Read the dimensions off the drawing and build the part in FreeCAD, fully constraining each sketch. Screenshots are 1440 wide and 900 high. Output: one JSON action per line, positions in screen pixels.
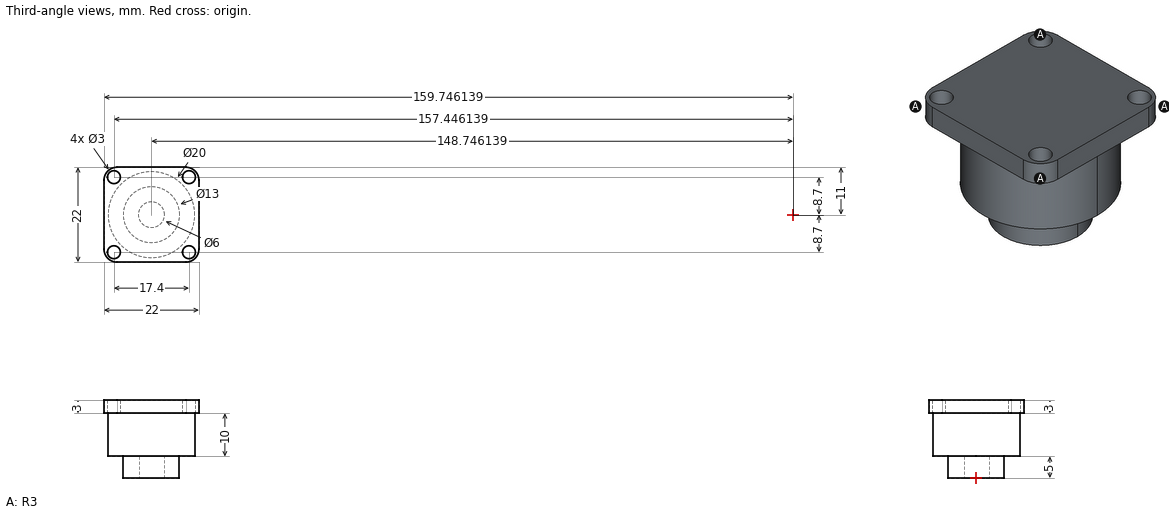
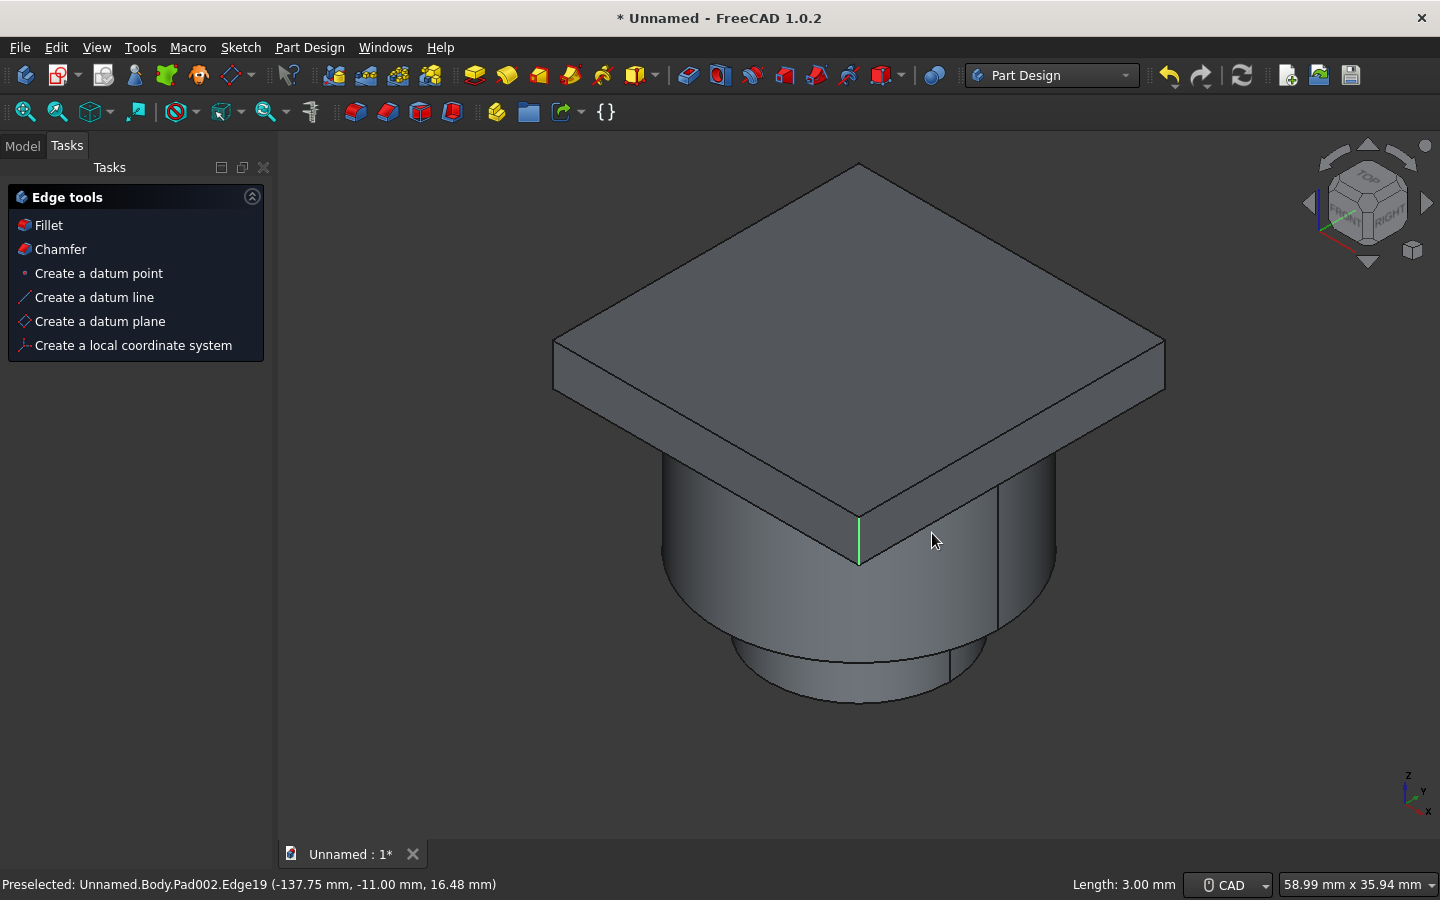
{"action": "key", "text": "2"}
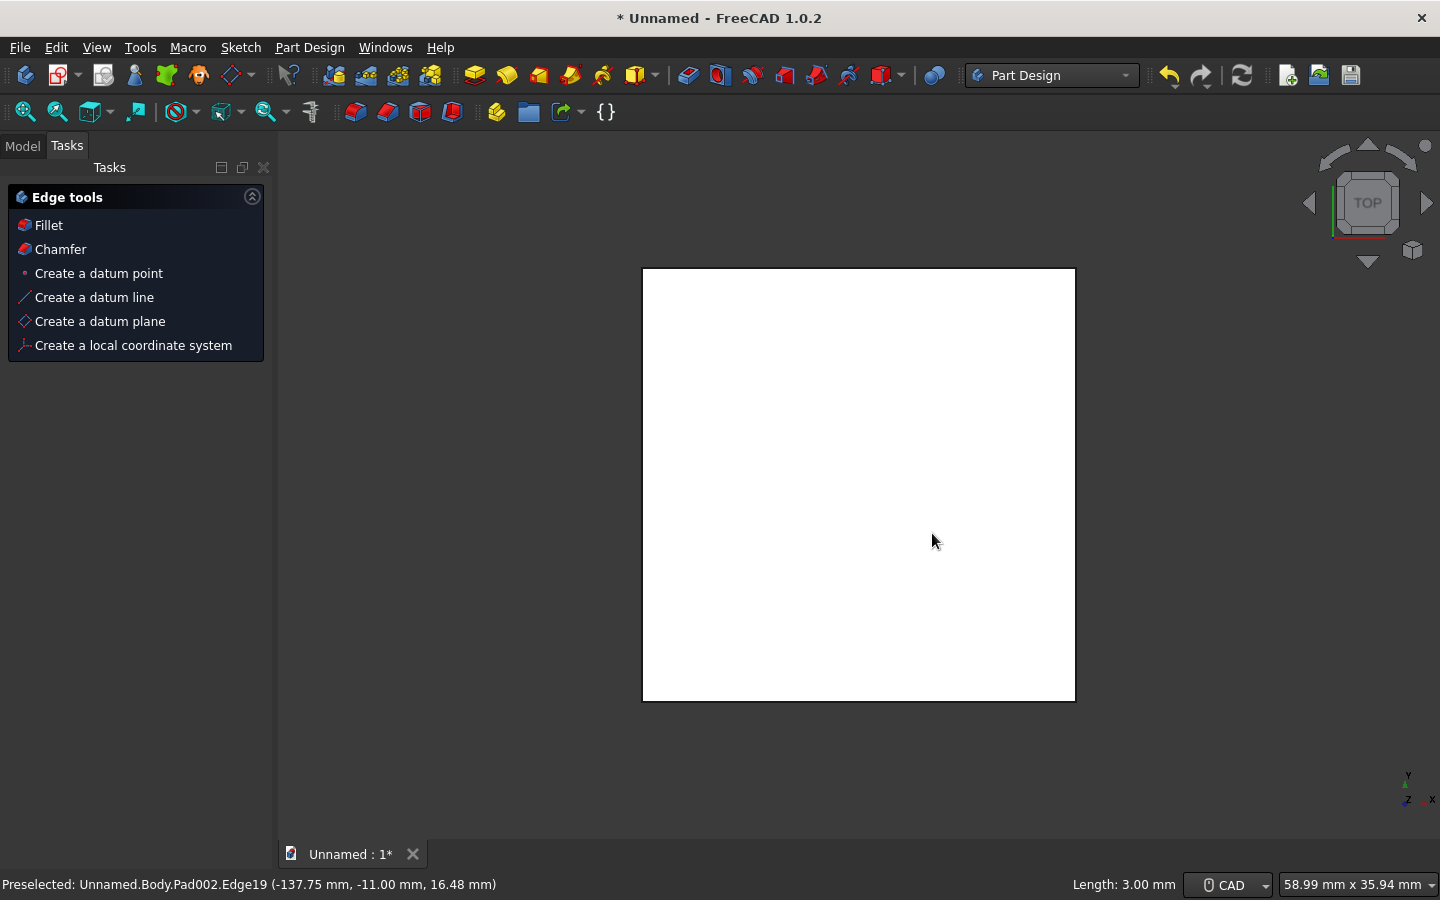
{"action": "key", "text": "1"}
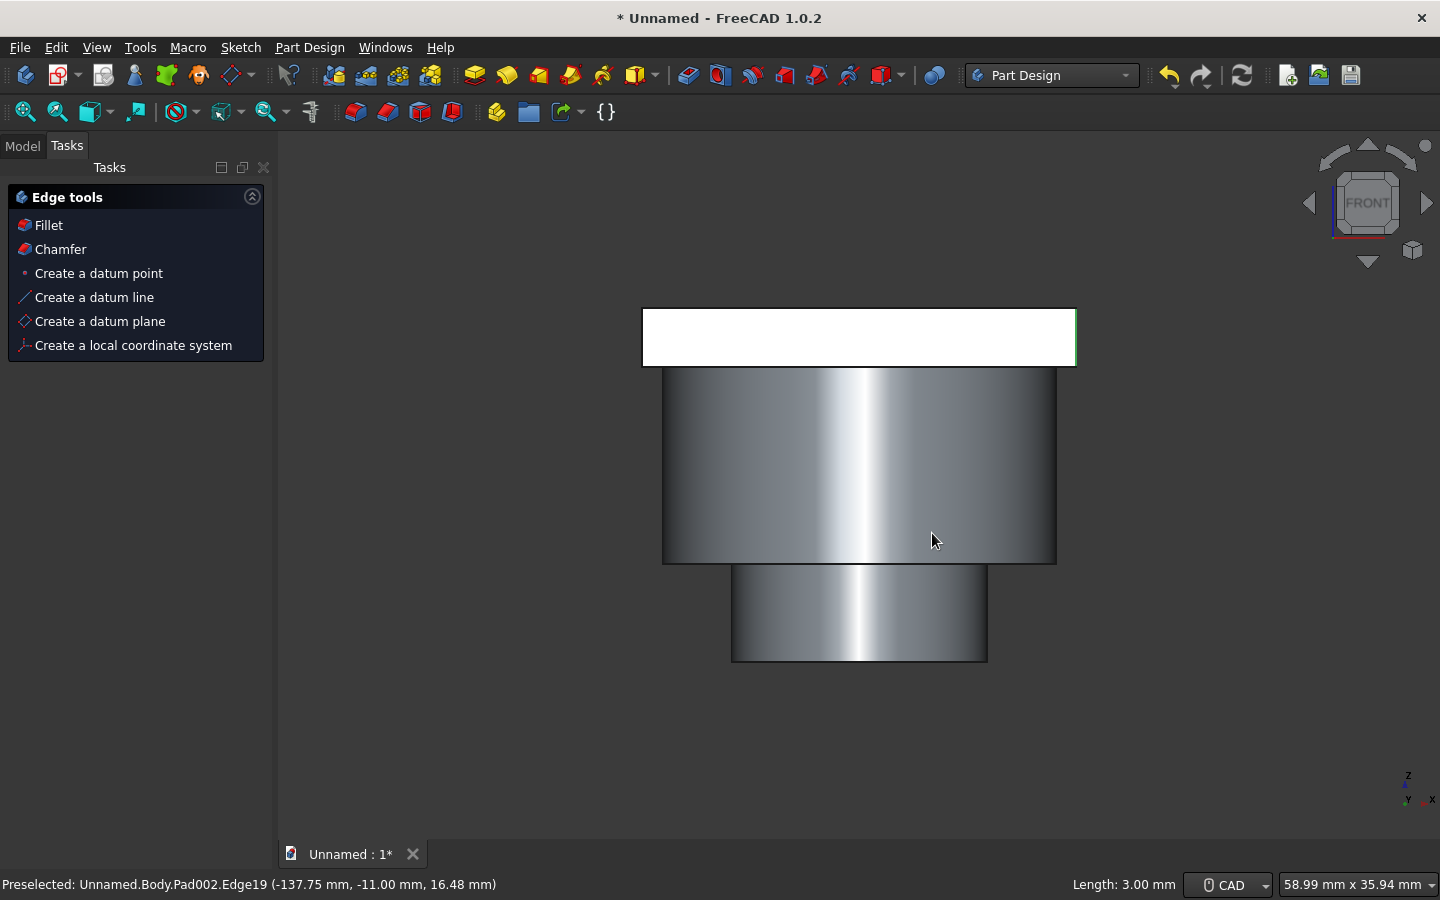
{"action": "left_click", "coordinate": [642, 336], "text": "ctrl"}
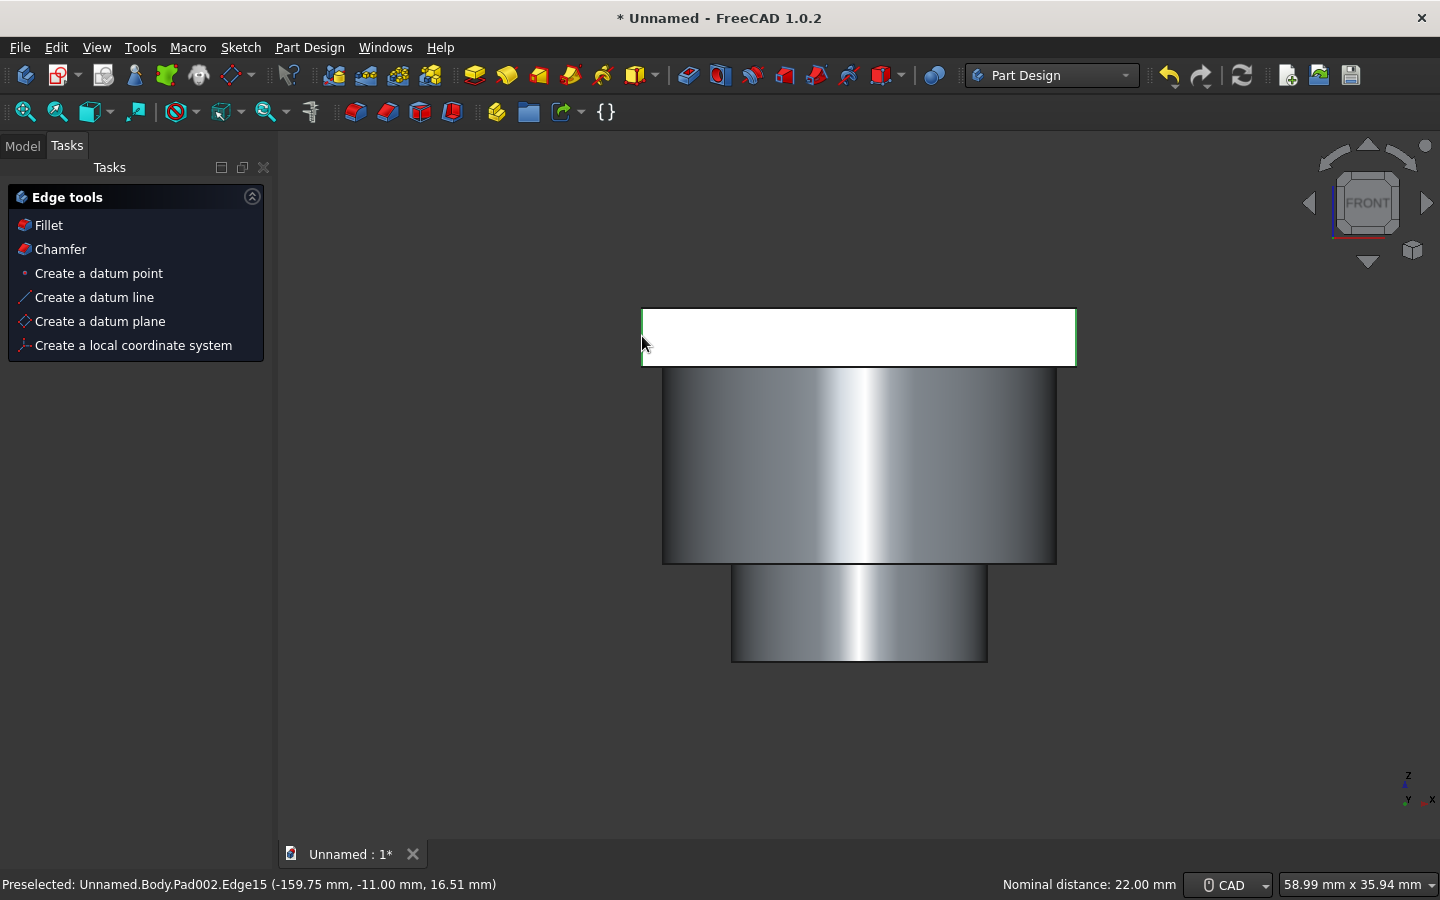
{"action": "key", "text": "3"}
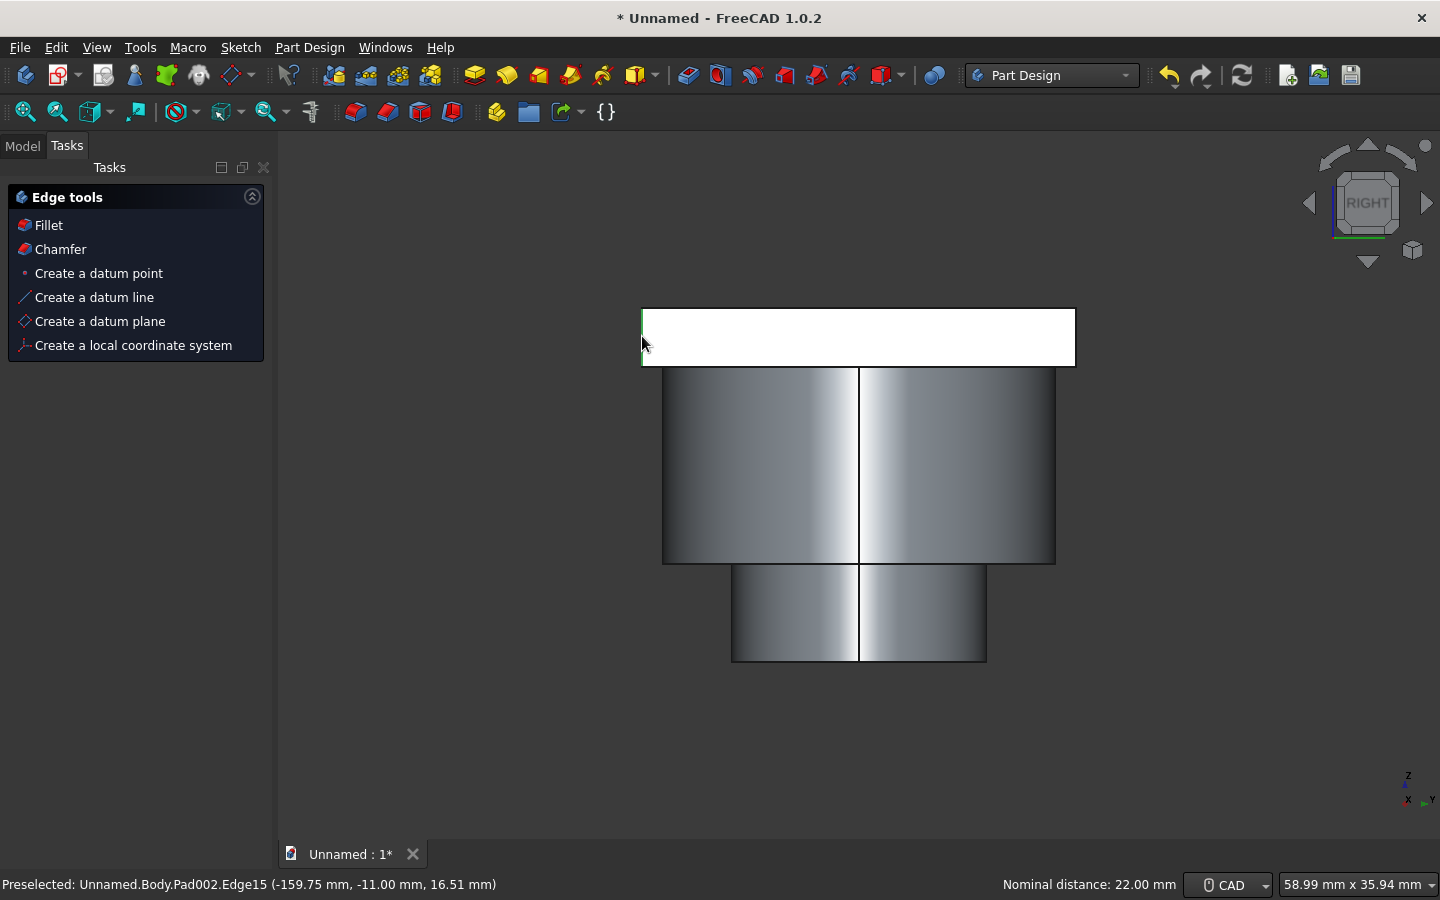
{"action": "left_click", "coordinate": [1076, 336], "text": "ctrl"}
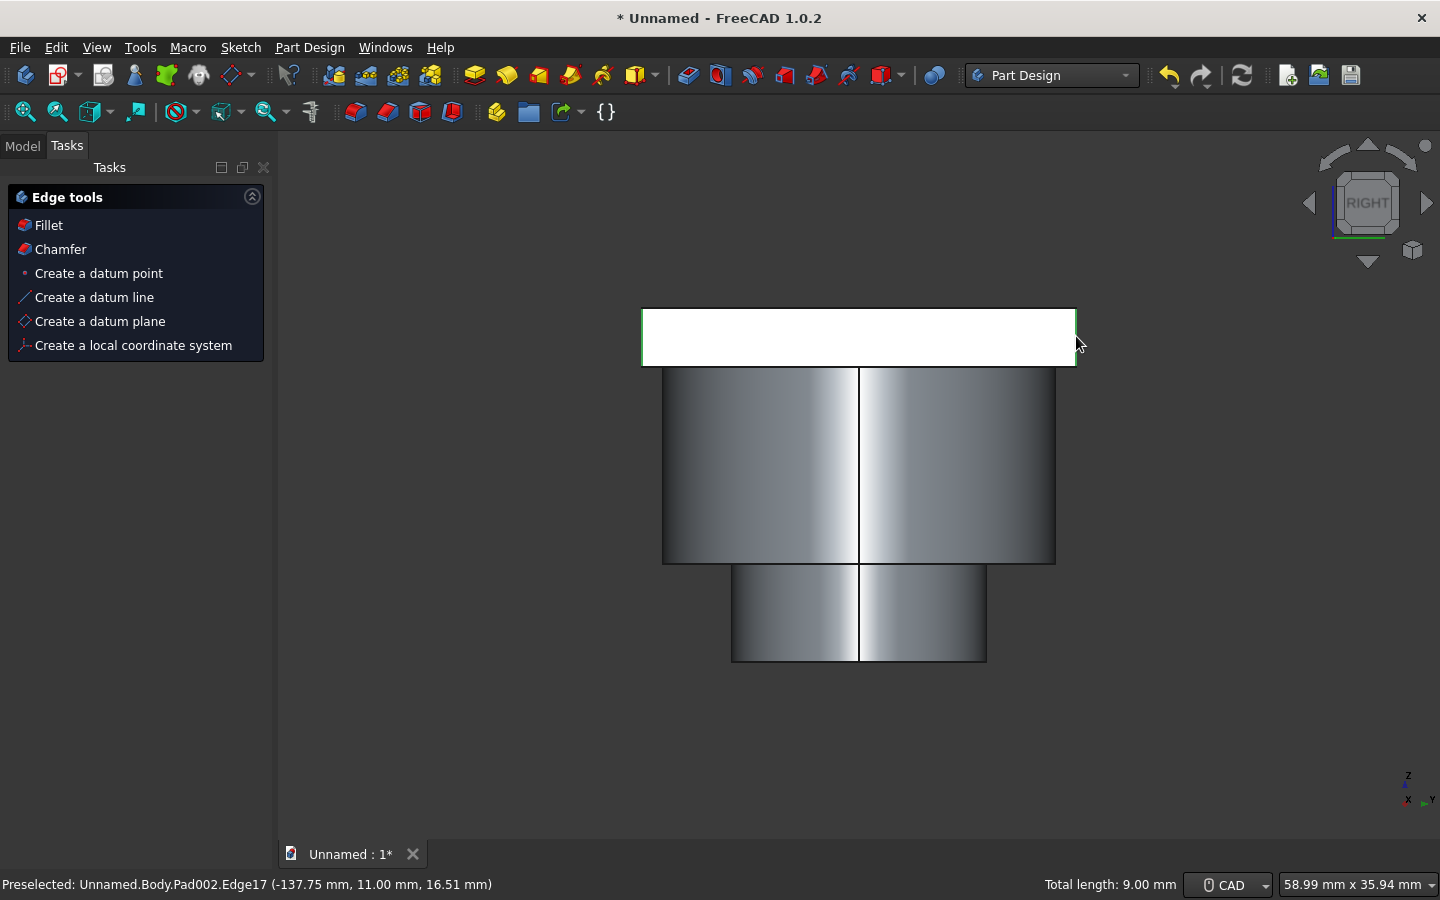
{"action": "key", "text": "5"}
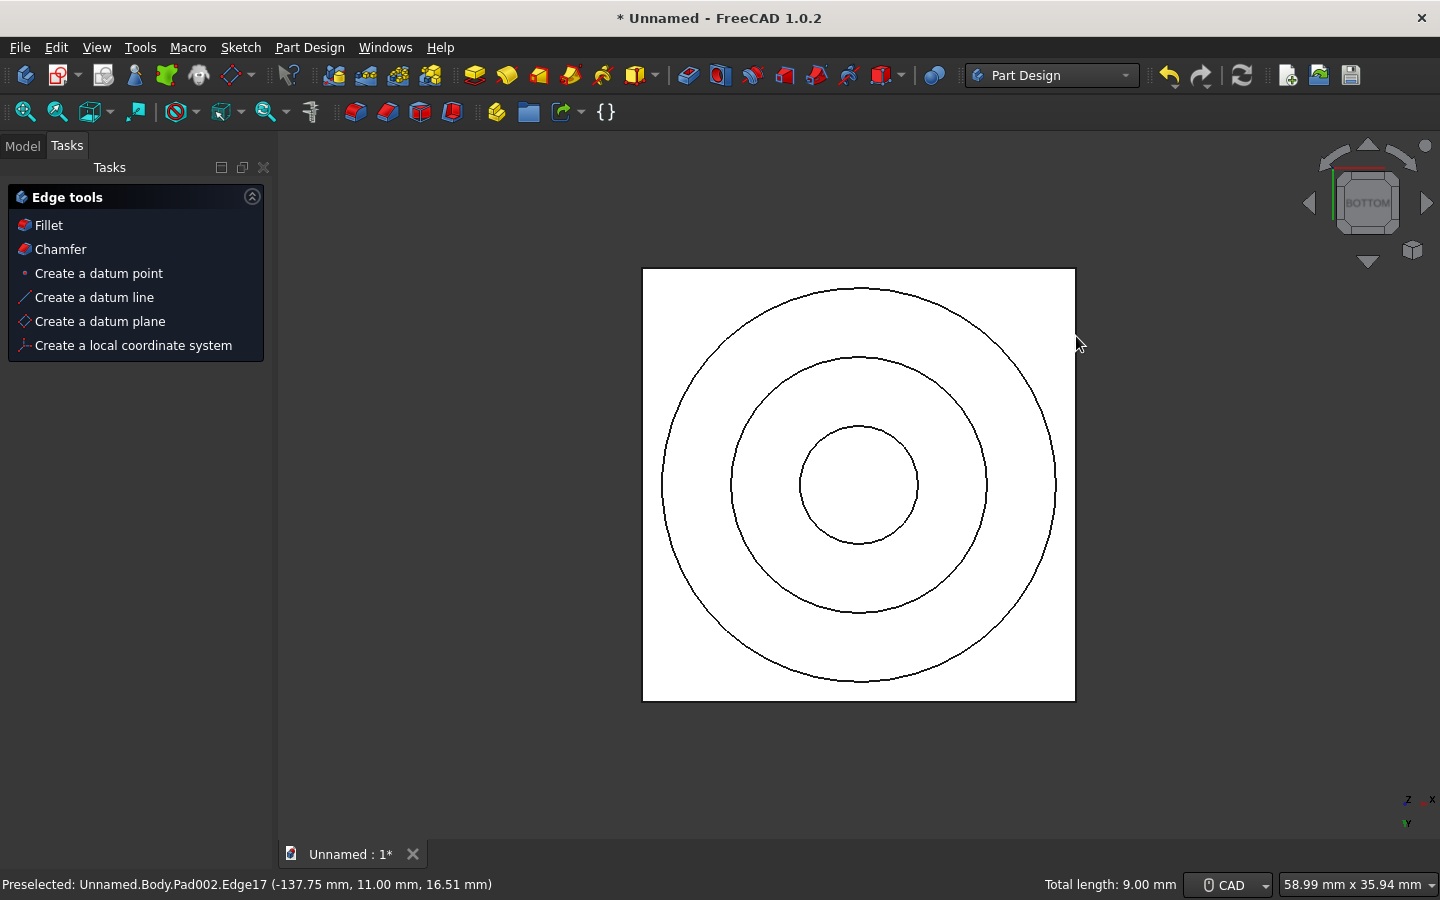
{"action": "key", "text": "4"}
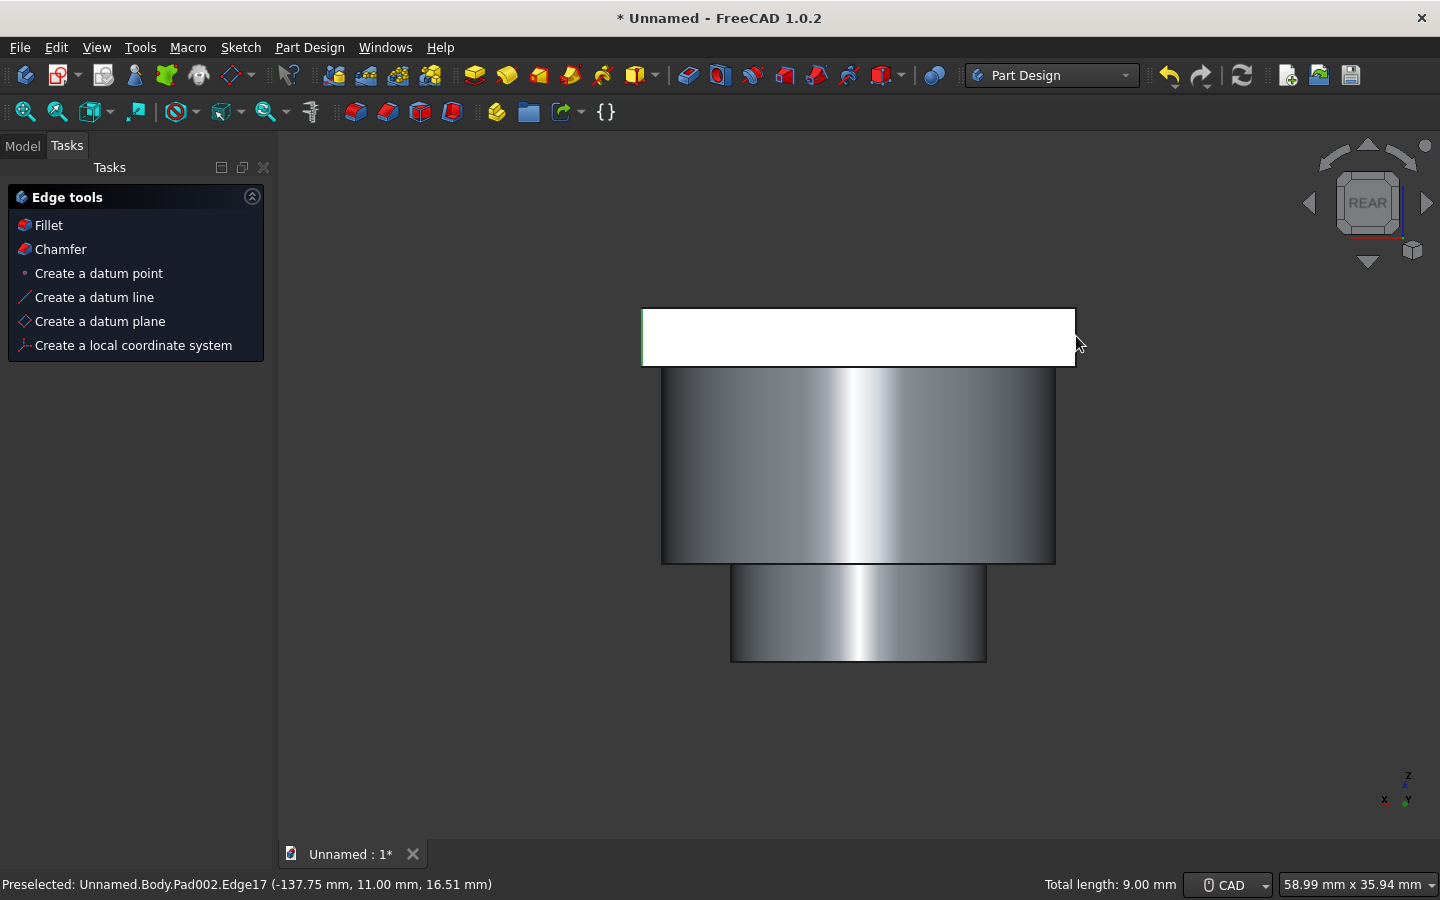
{"action": "left_click", "coordinate": [1076, 336], "text": "ctrl"}